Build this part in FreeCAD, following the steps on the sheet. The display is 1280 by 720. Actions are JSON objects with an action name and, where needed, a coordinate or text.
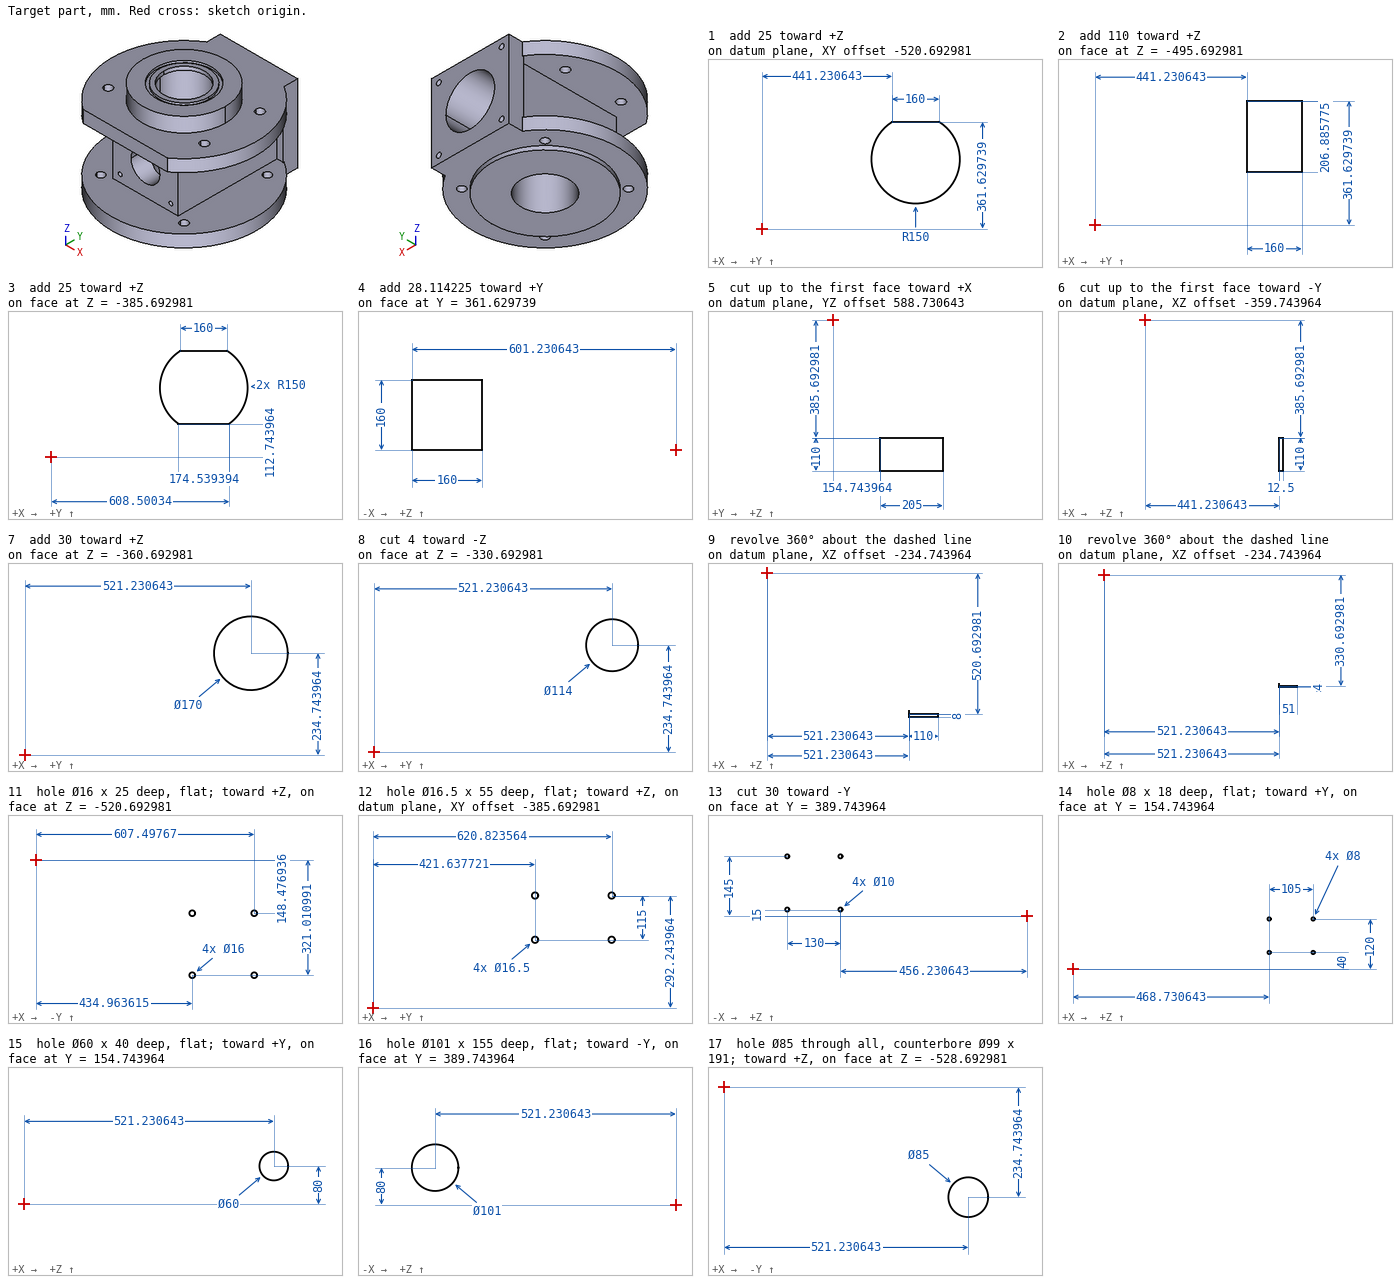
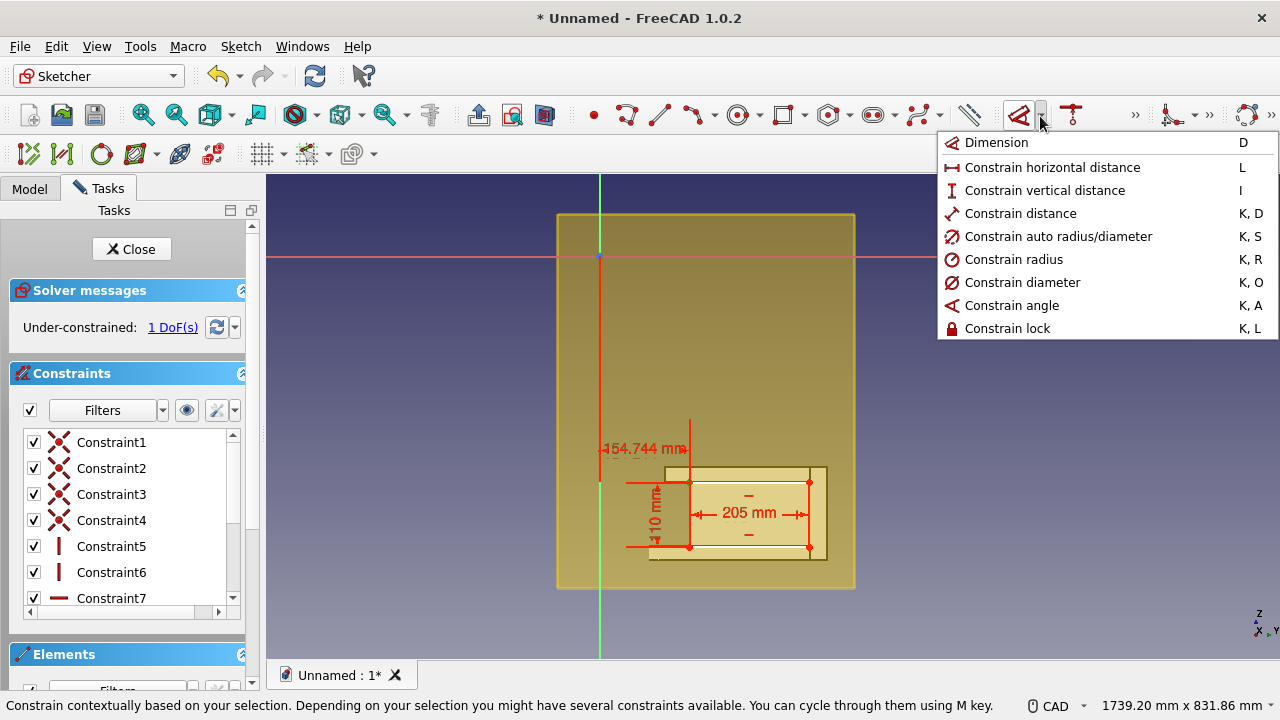
{"action": "left_click", "coordinate": [1108, 190]}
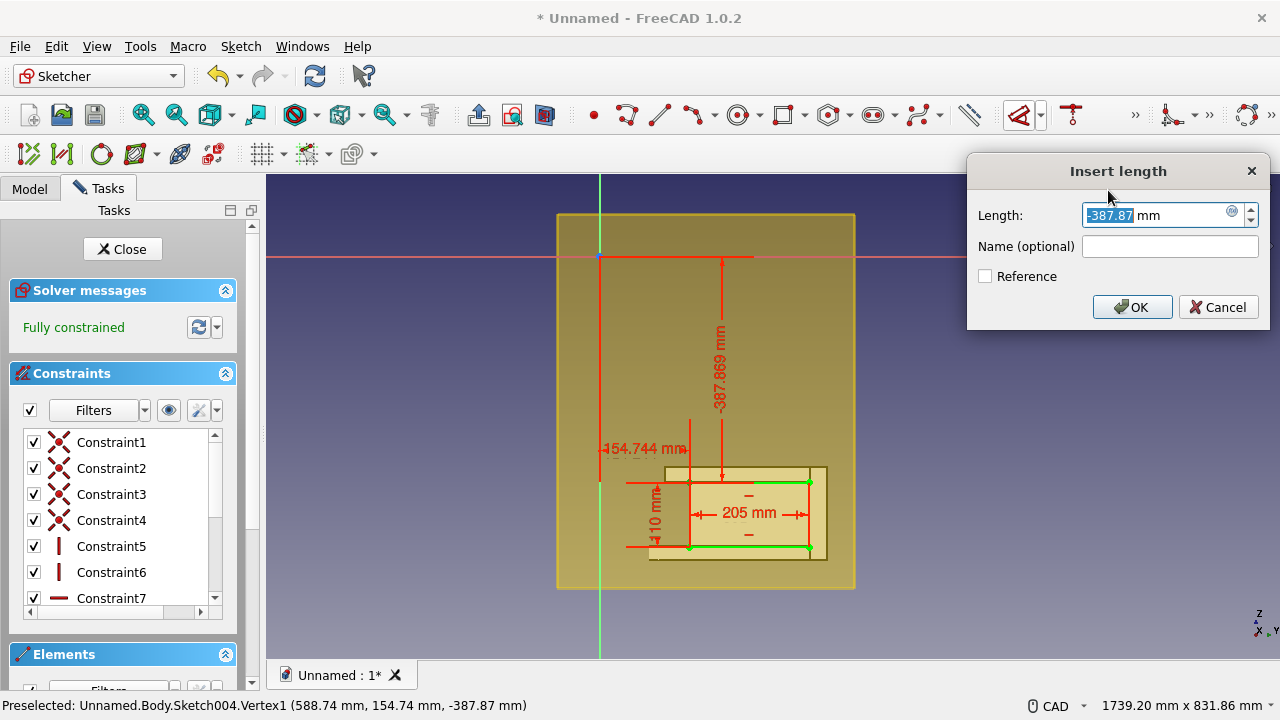
{"action": "type", "text": "-385.692981"}
{"action": "key", "text": "Return"}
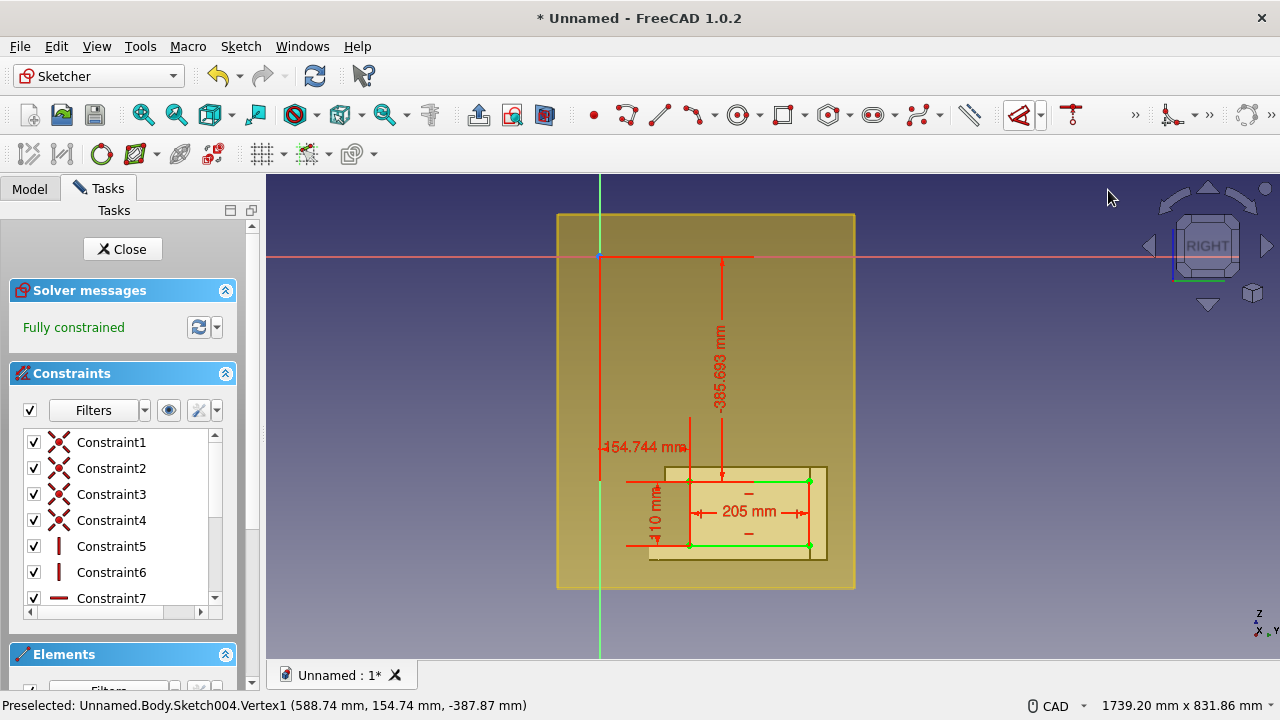
{"action": "left_click", "coordinate": [123, 249]}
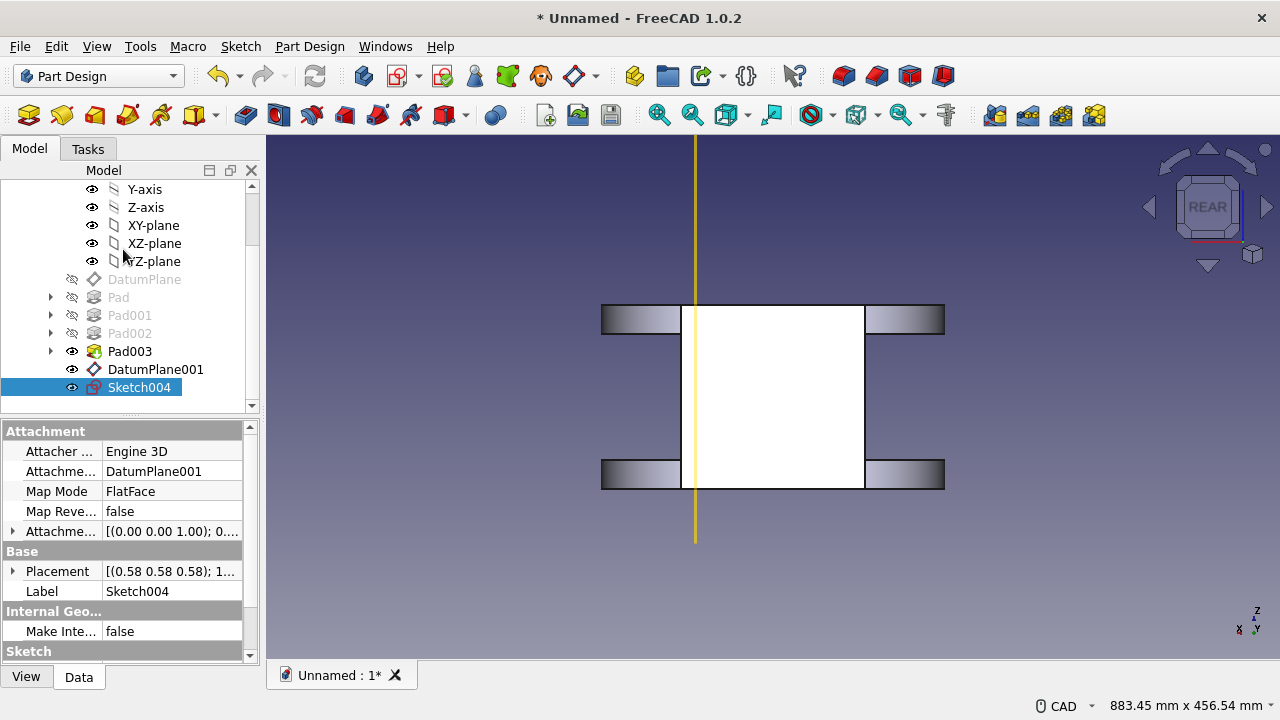
{"action": "left_click", "coordinate": [246, 116]}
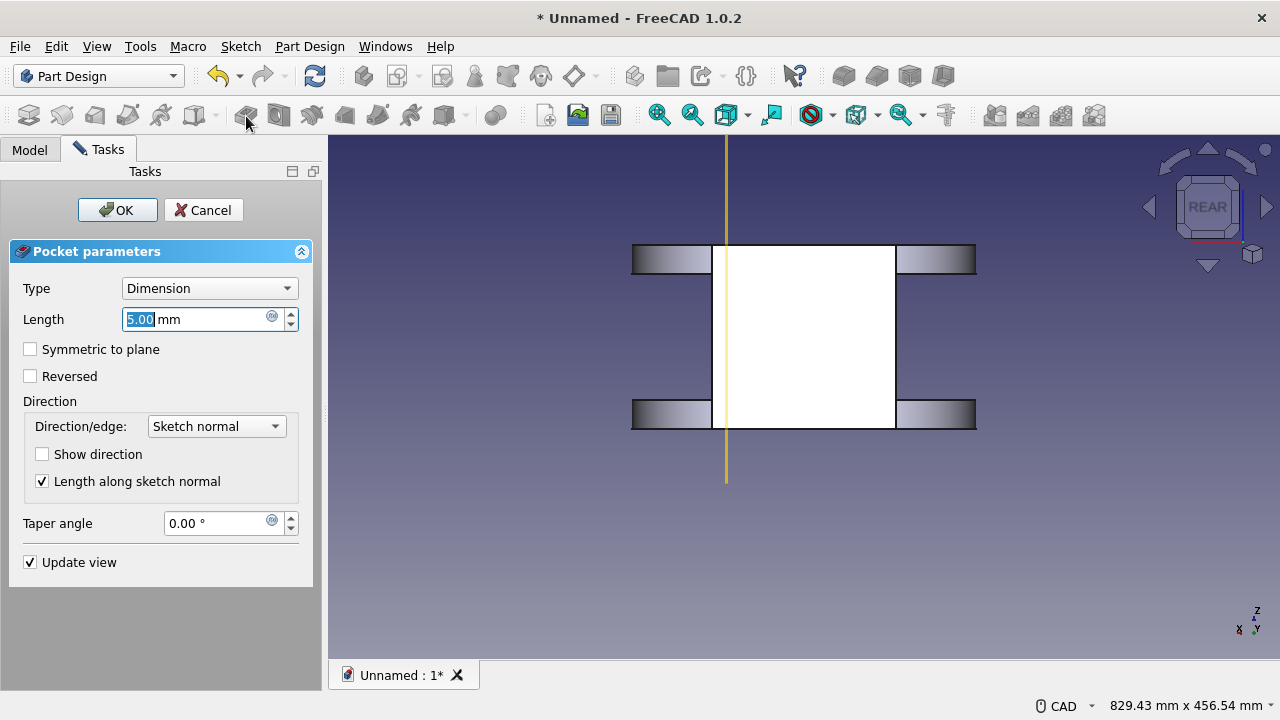
{"action": "left_click", "coordinate": [210, 288]}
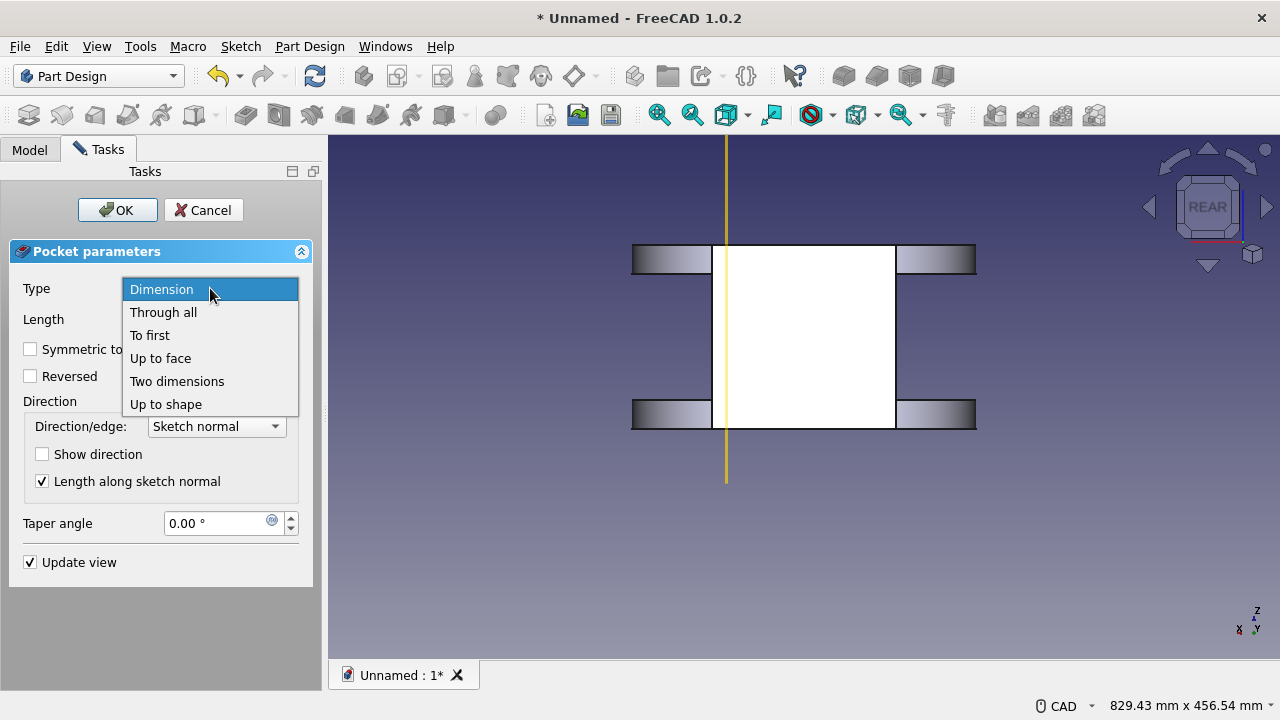
{"action": "left_click", "coordinate": [208, 336]}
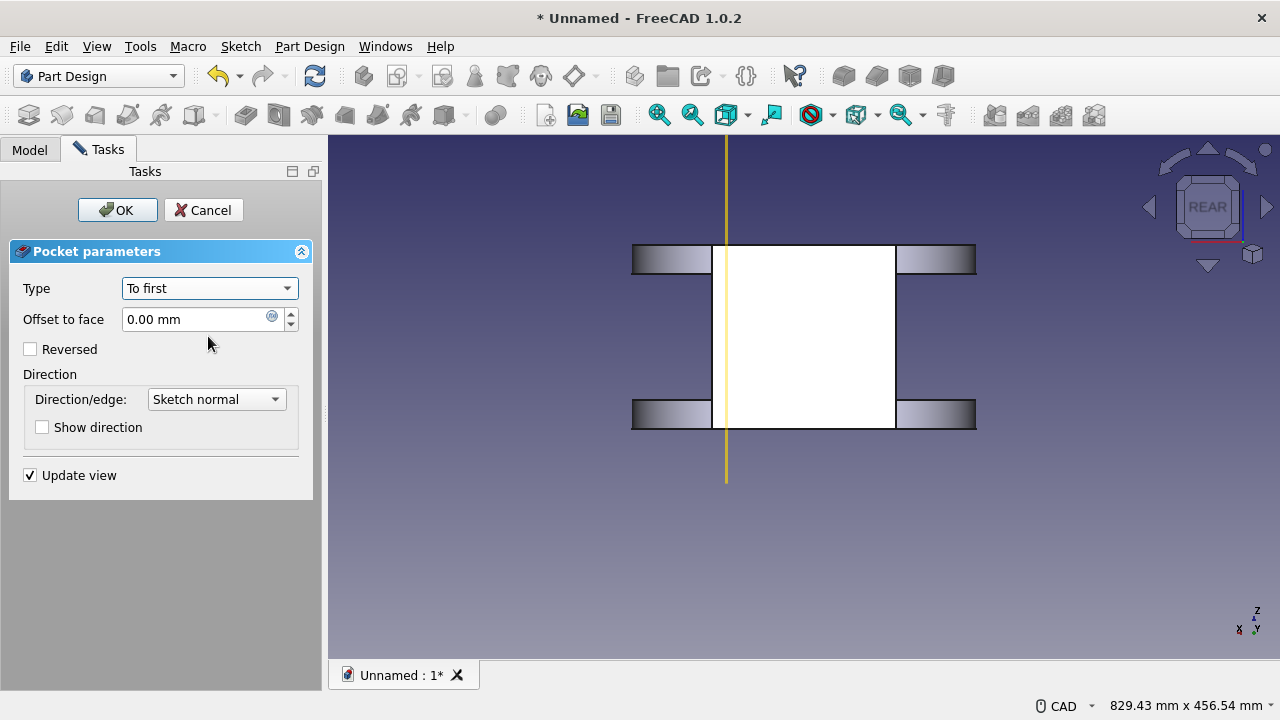
{"action": "left_click", "coordinate": [31, 349]}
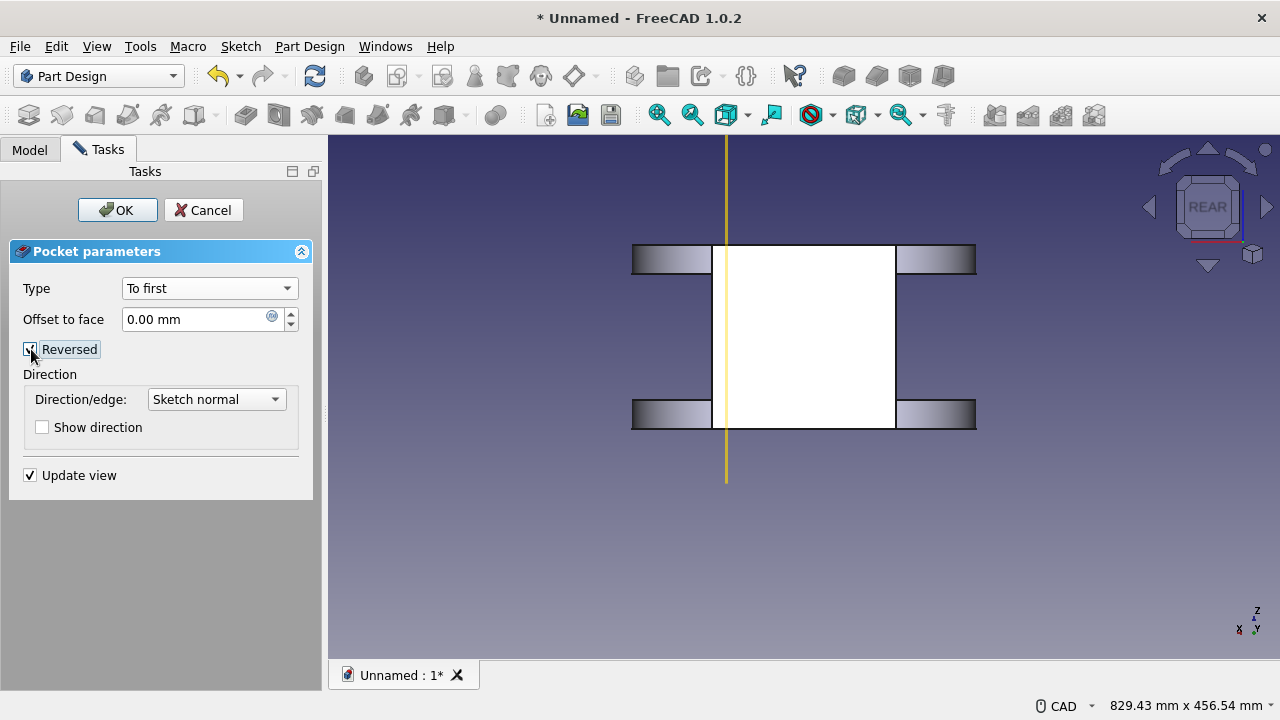
{"action": "left_click", "coordinate": [118, 210]}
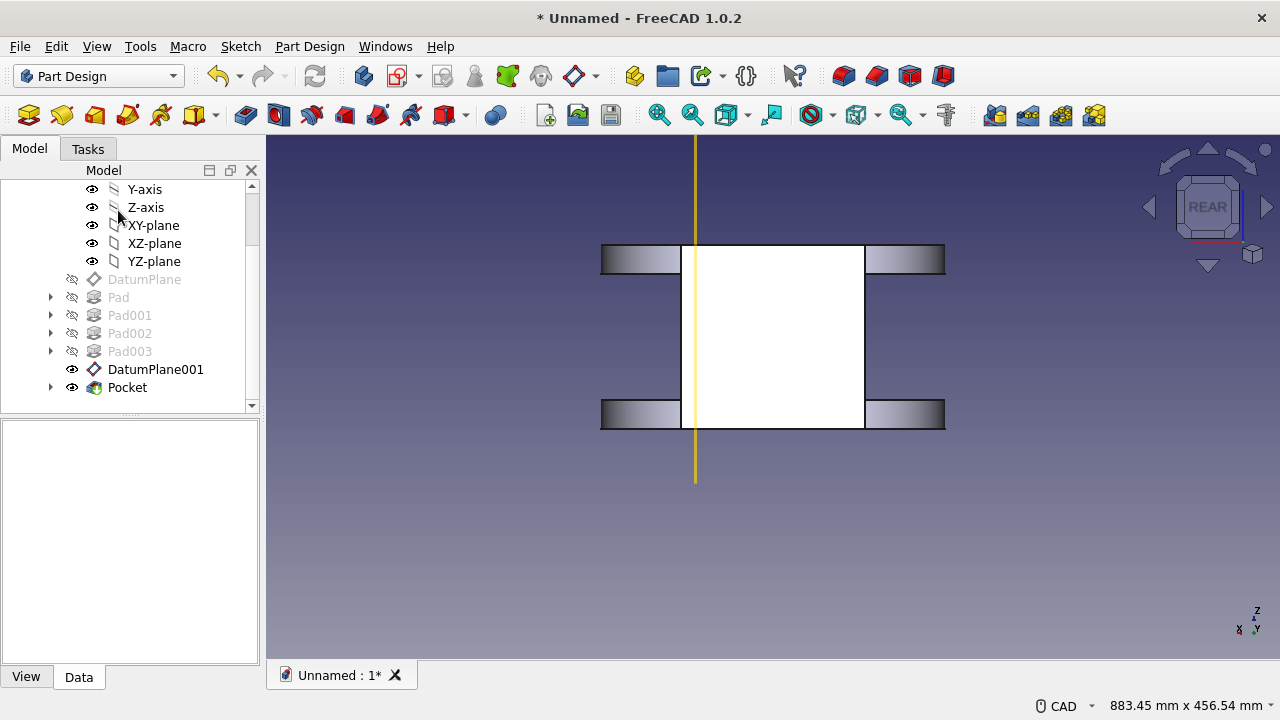
{"action": "left_click", "coordinate": [117, 369]}
{"action": "key", "text": "space"}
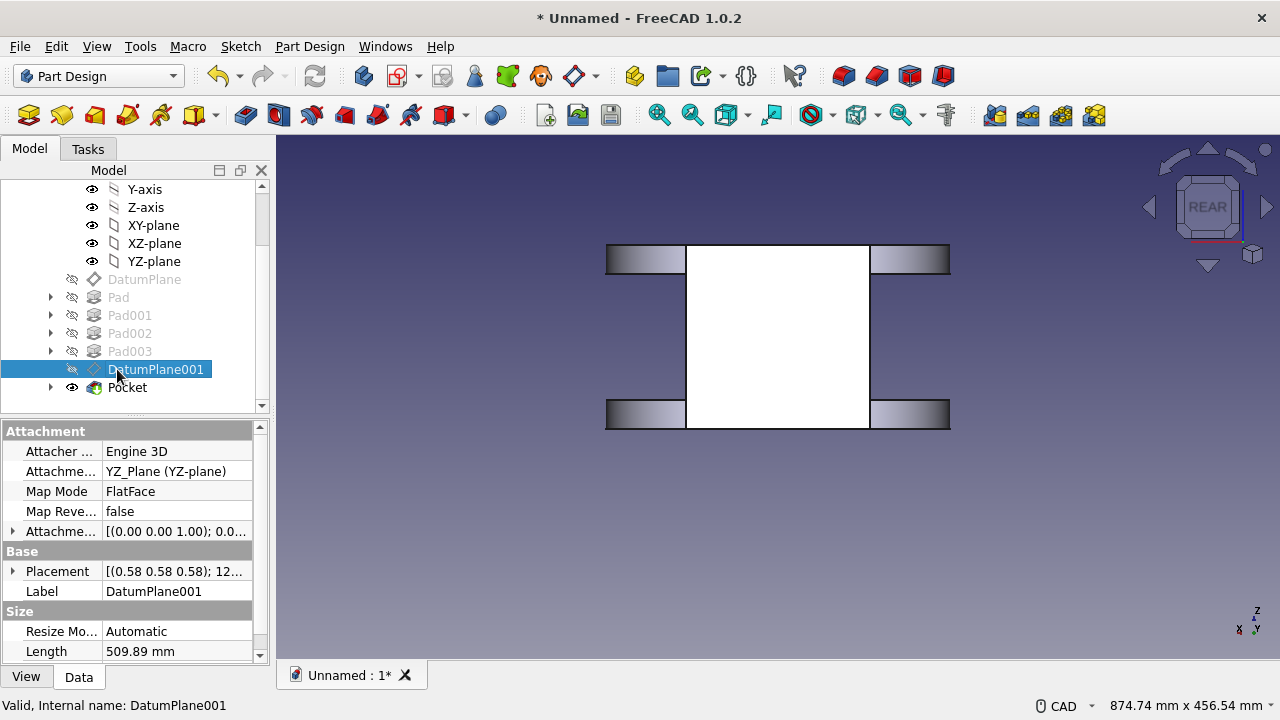
{"action": "left_click", "coordinate": [660, 116]}